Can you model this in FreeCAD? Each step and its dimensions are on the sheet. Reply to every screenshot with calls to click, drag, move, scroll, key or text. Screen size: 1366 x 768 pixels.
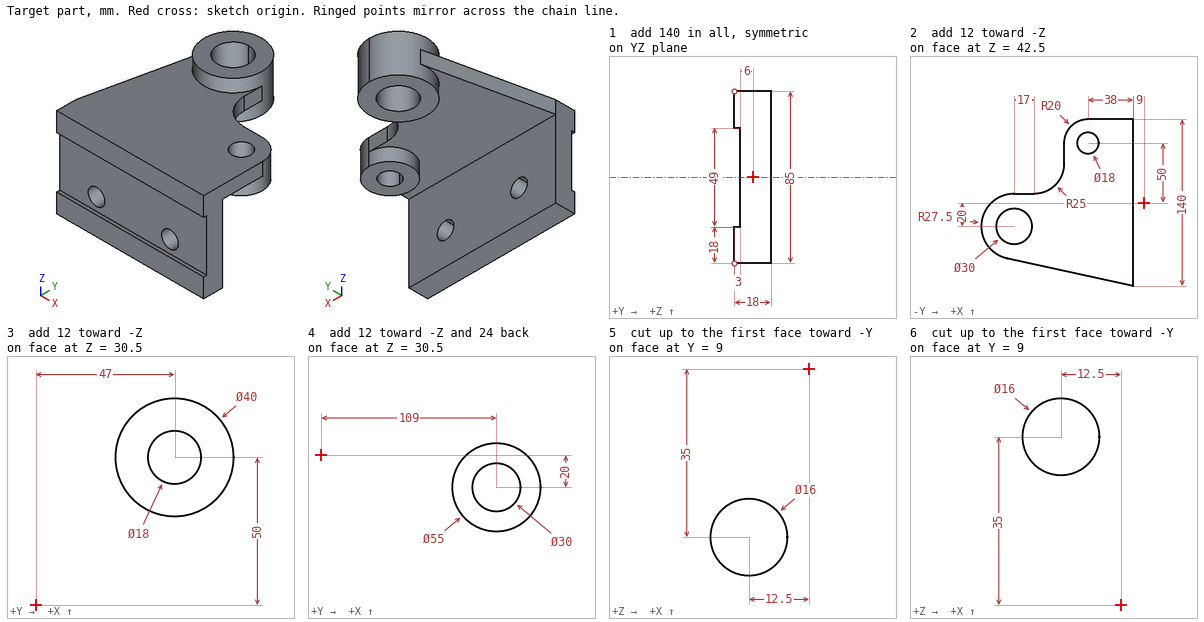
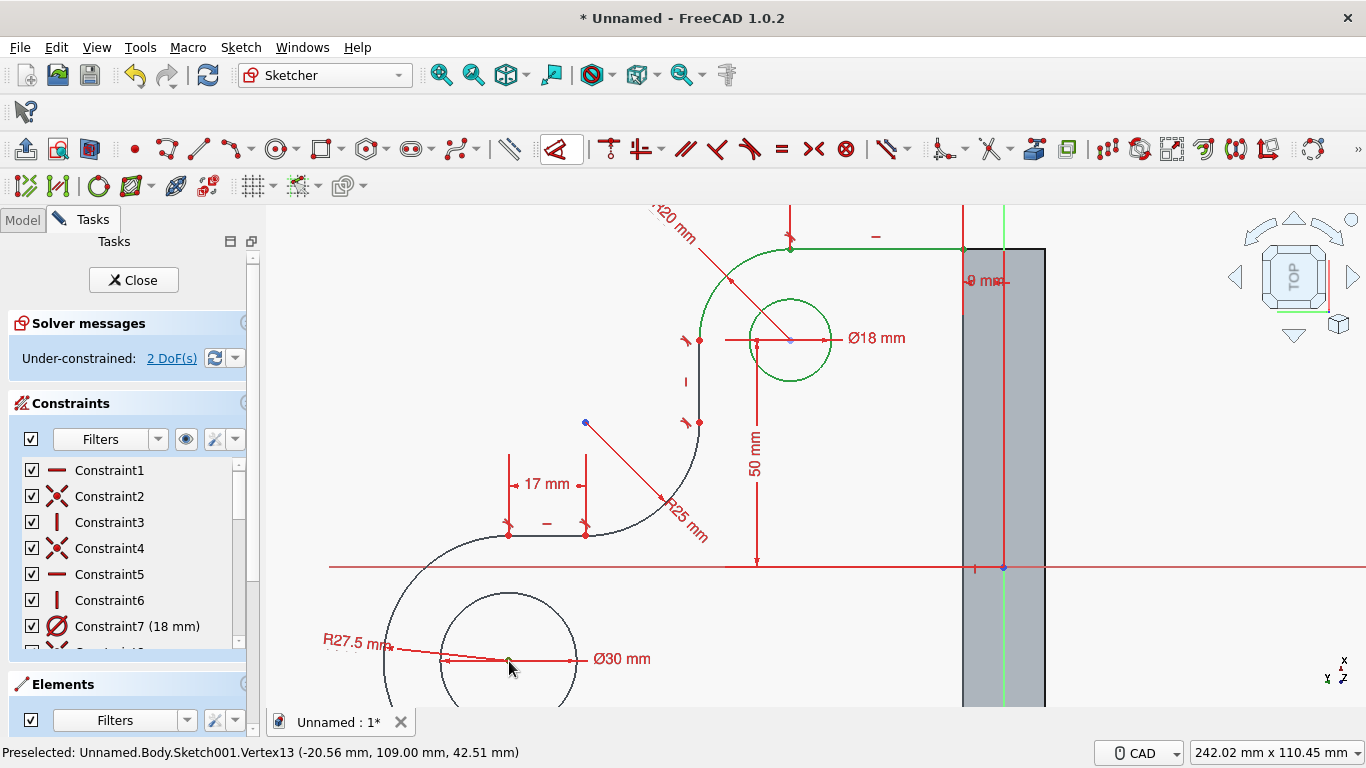
key(i)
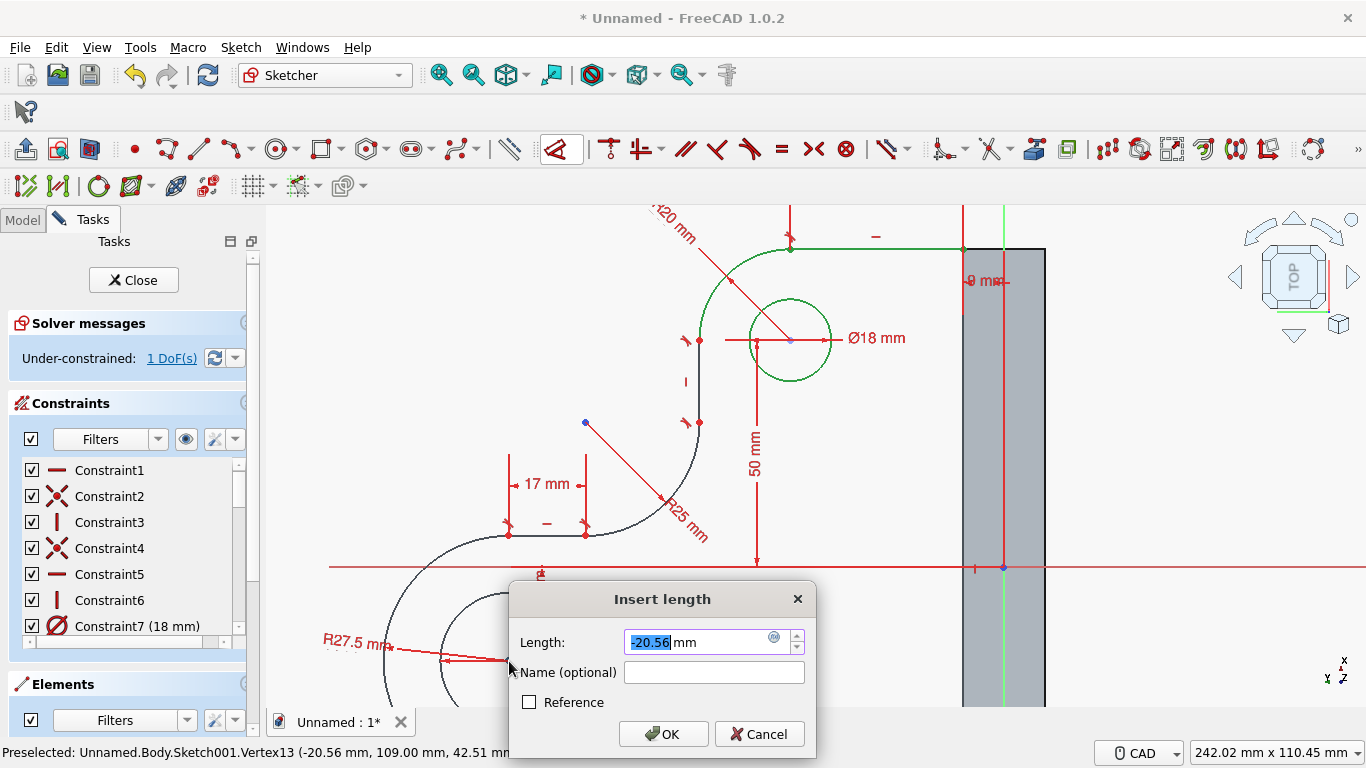
text(-20)
key(Return)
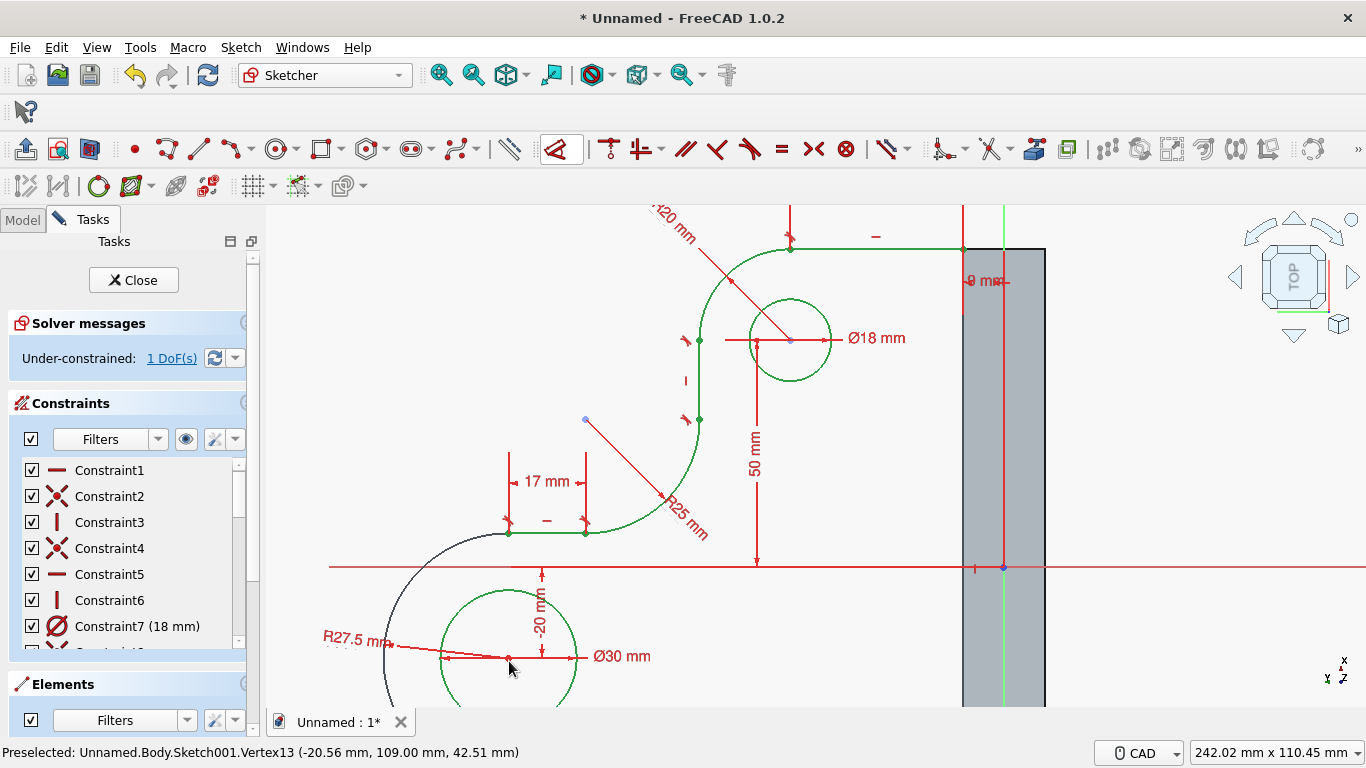
click(963, 441)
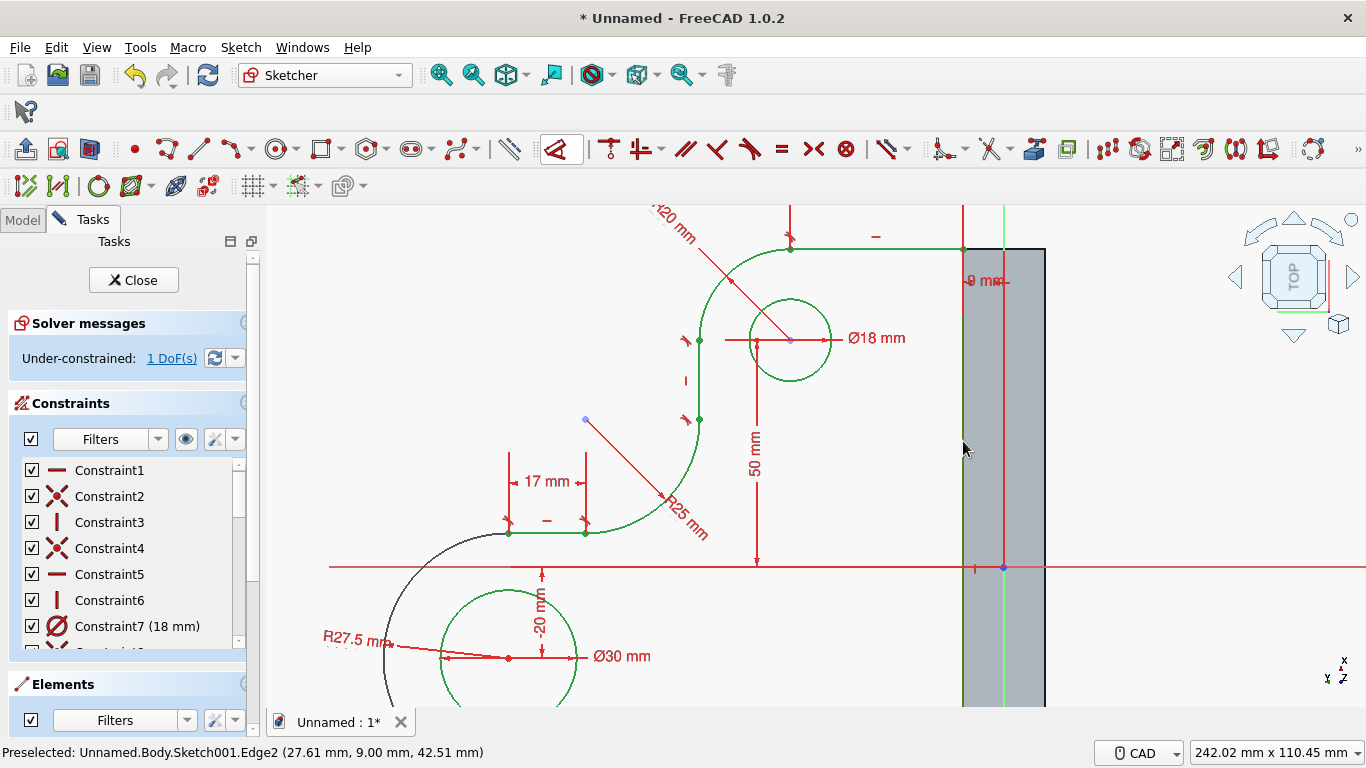
key(i)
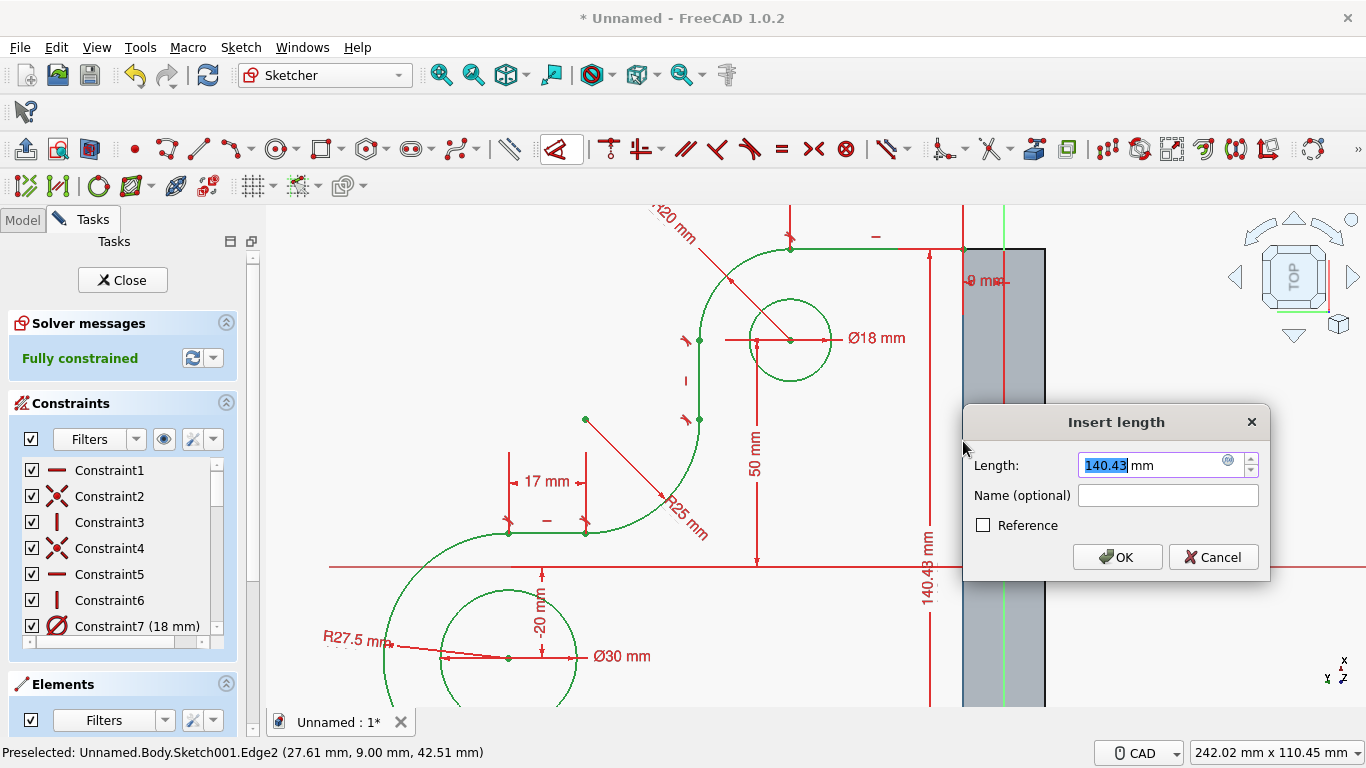
text(140)
key(Return)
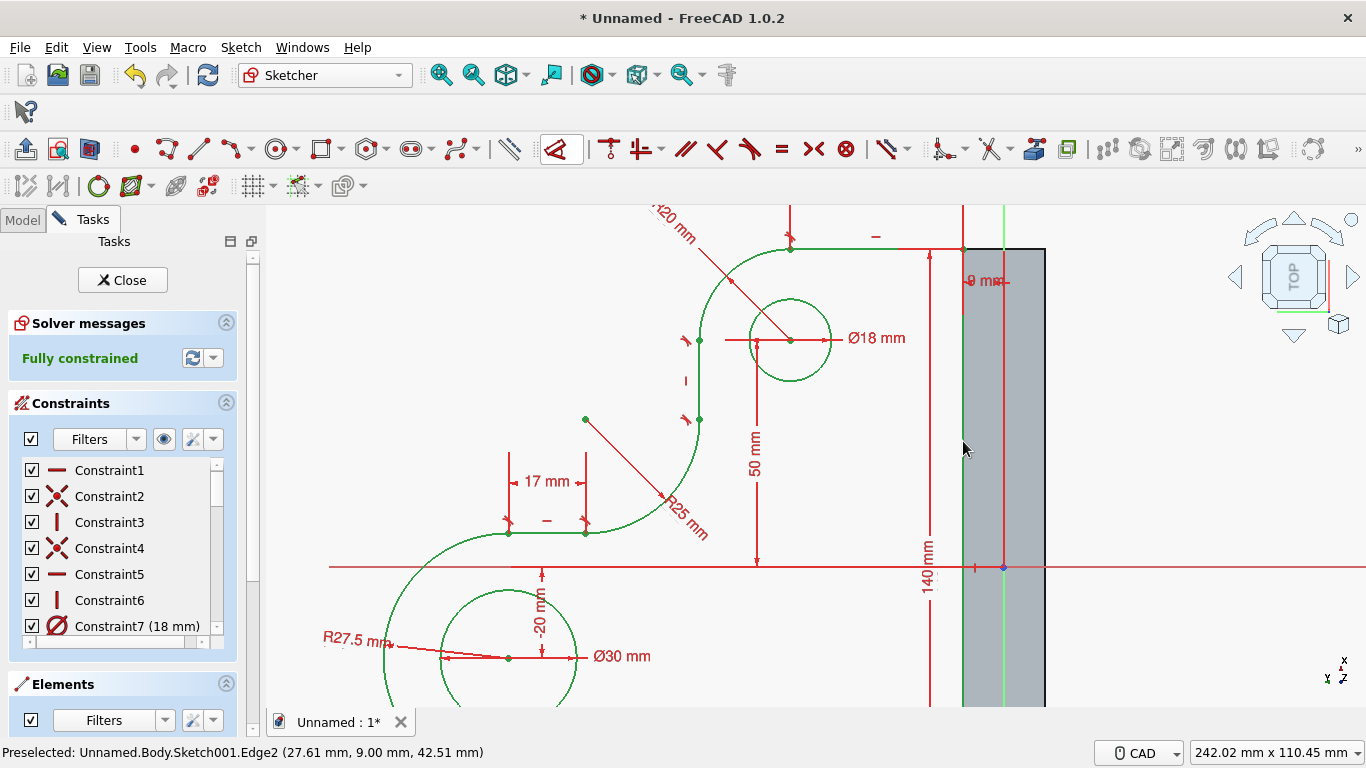
click(123, 280)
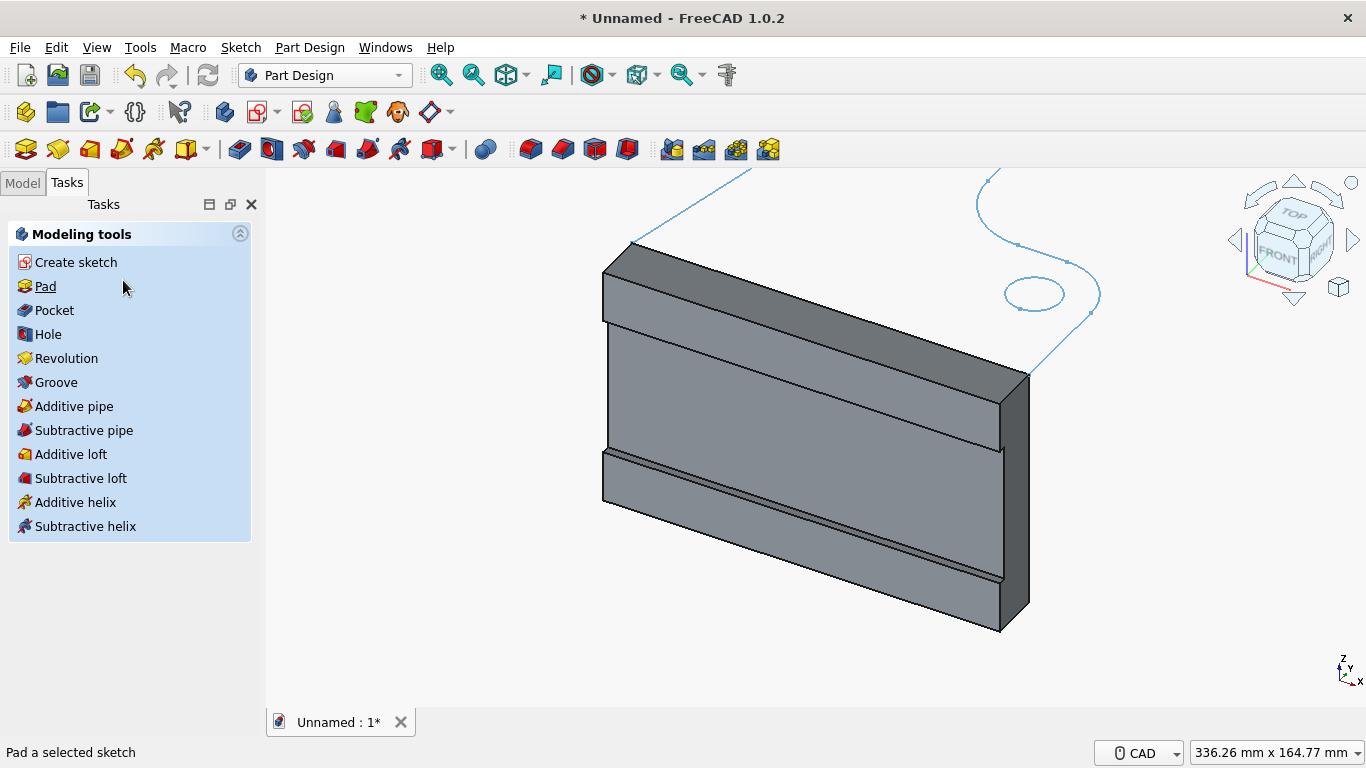
click(26, 150)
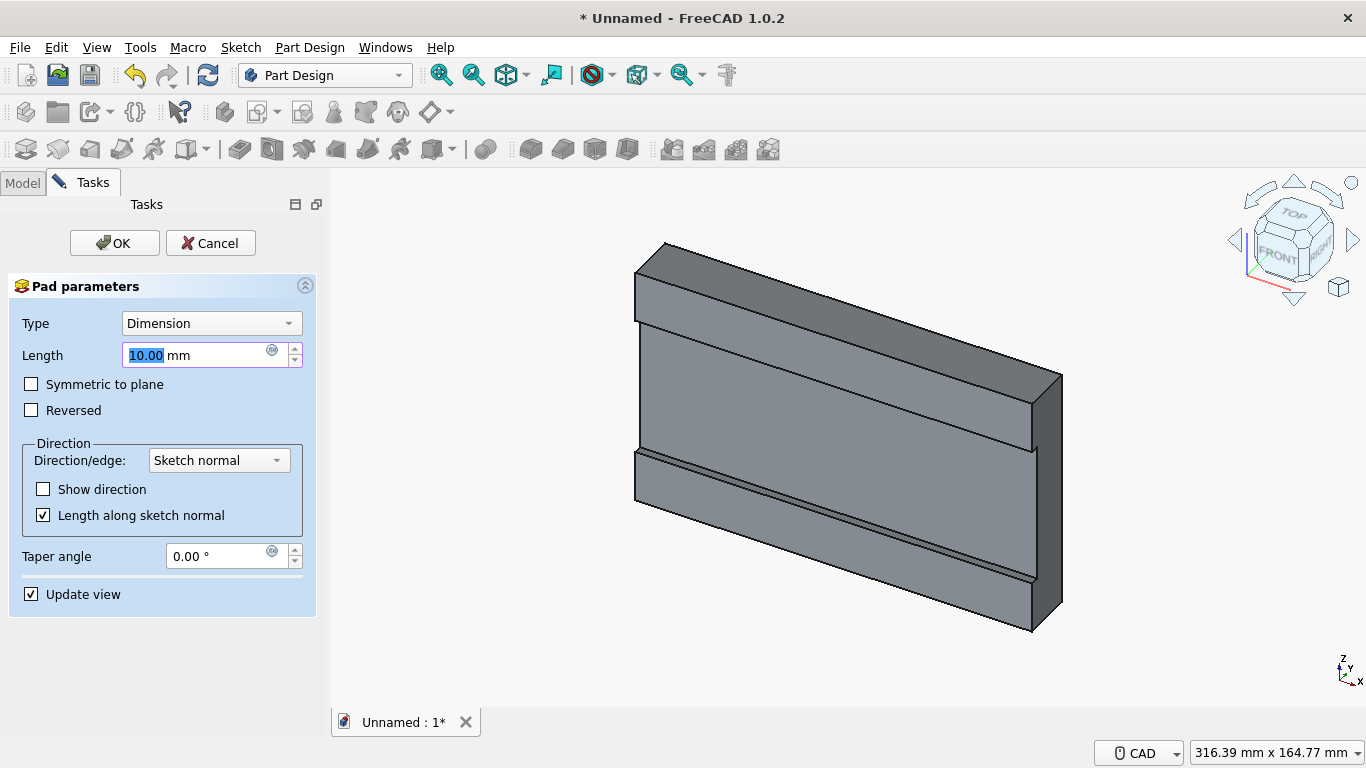
text(12)
key(Tab)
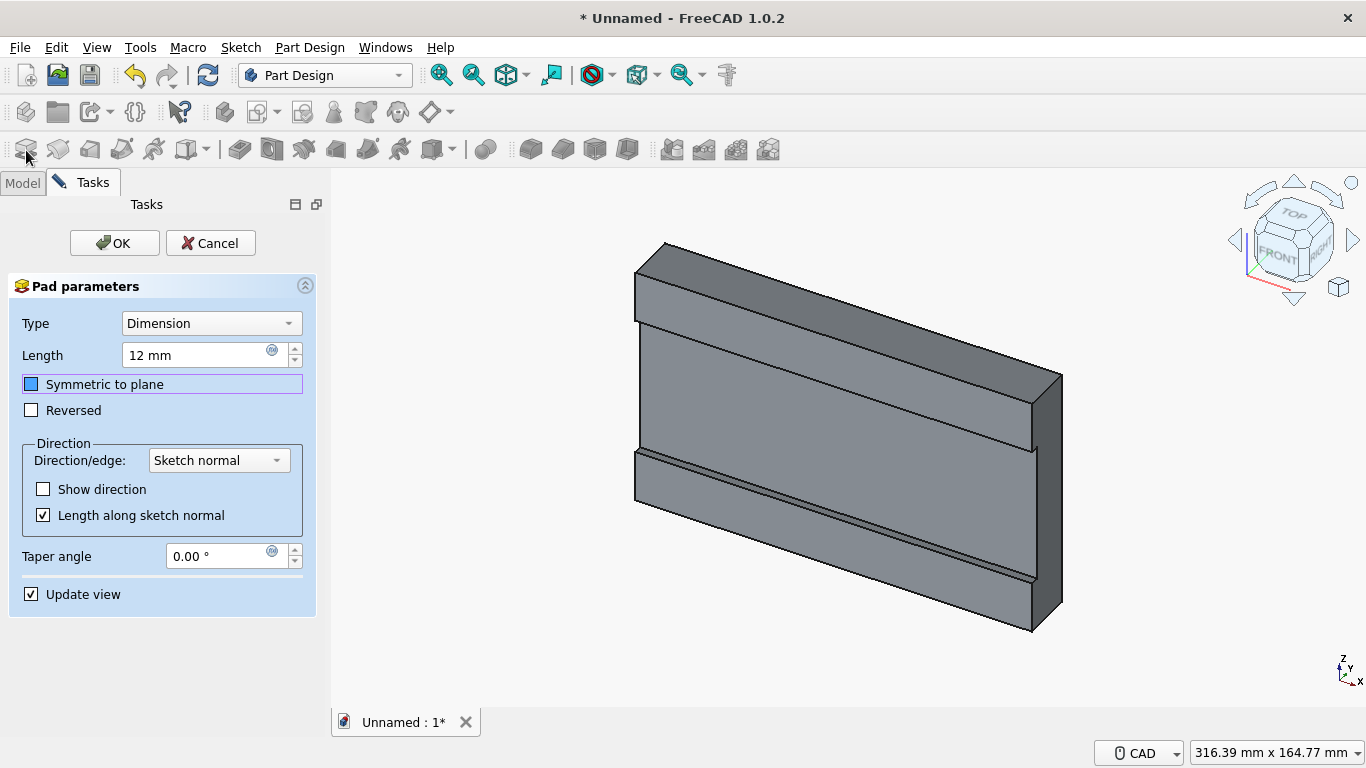
click(30, 410)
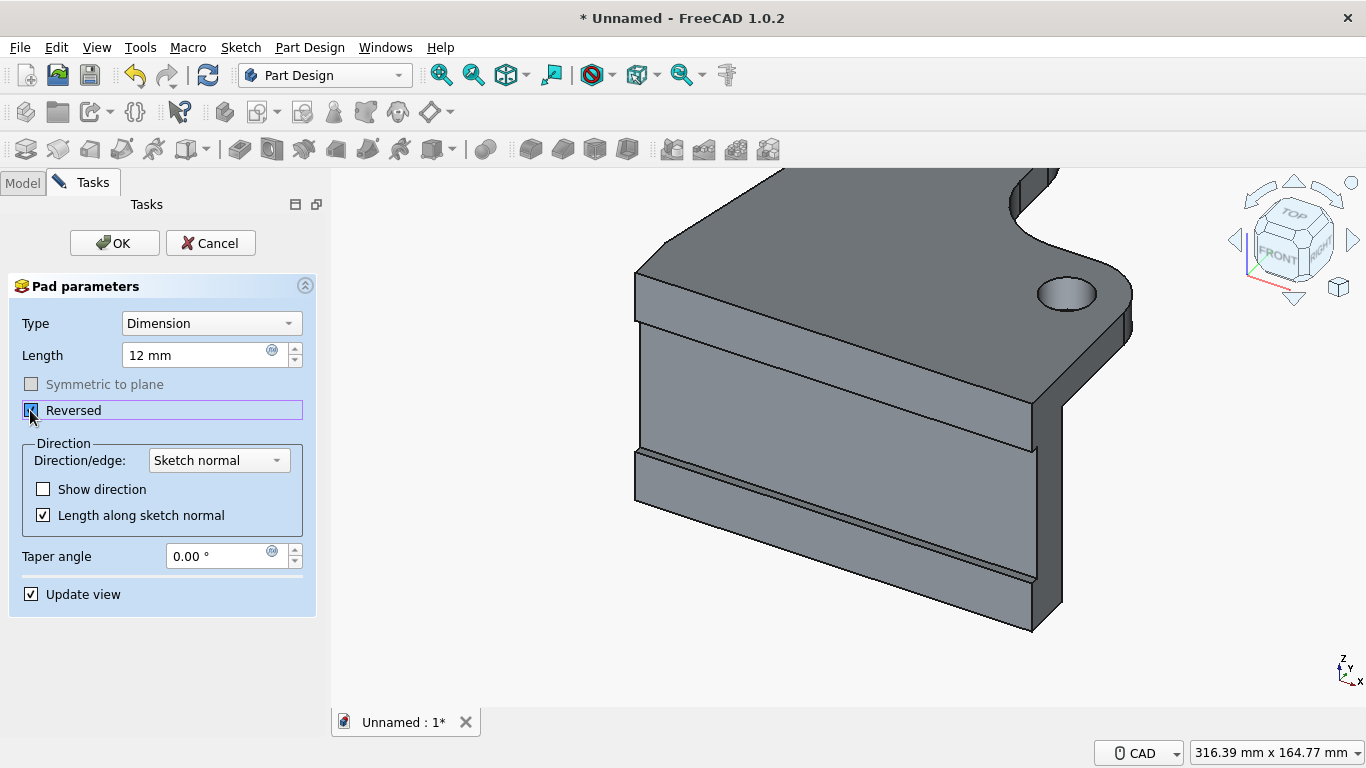
click(115, 243)